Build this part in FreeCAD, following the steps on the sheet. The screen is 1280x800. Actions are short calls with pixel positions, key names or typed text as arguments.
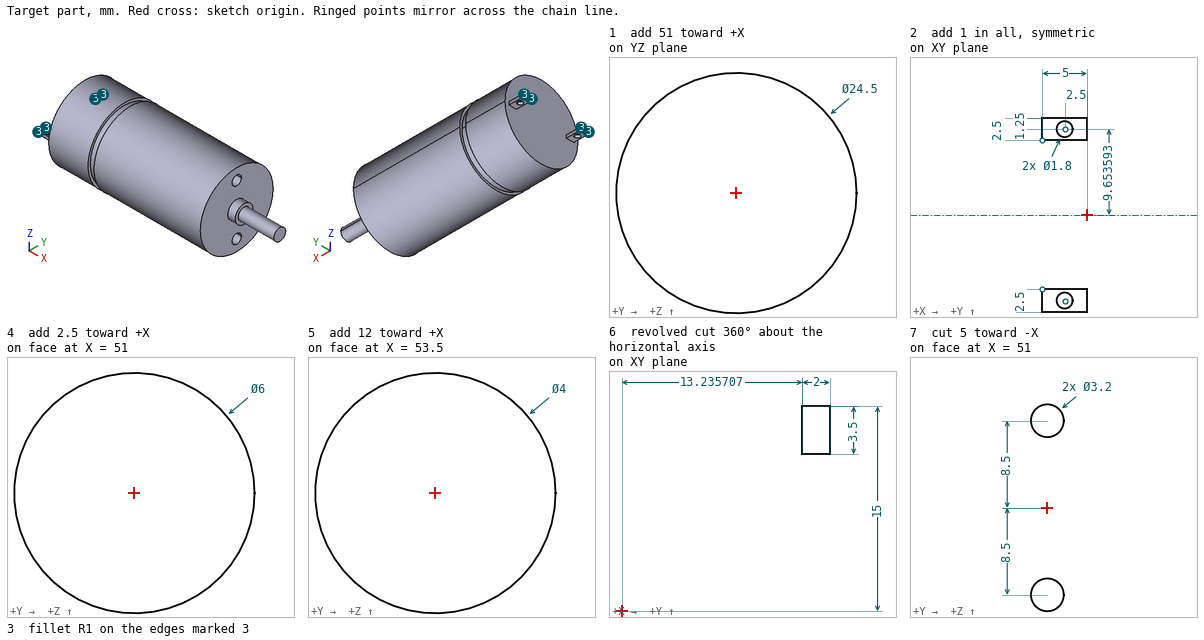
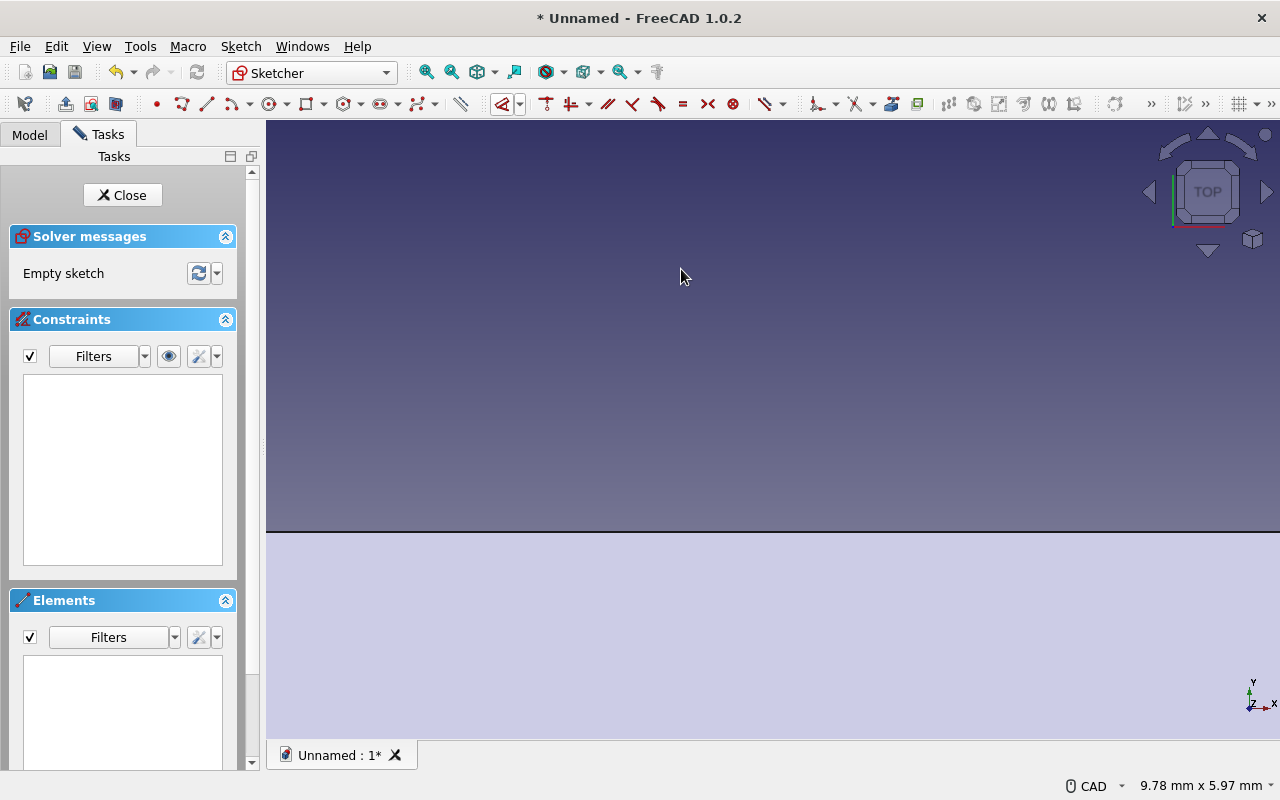
click(306, 104)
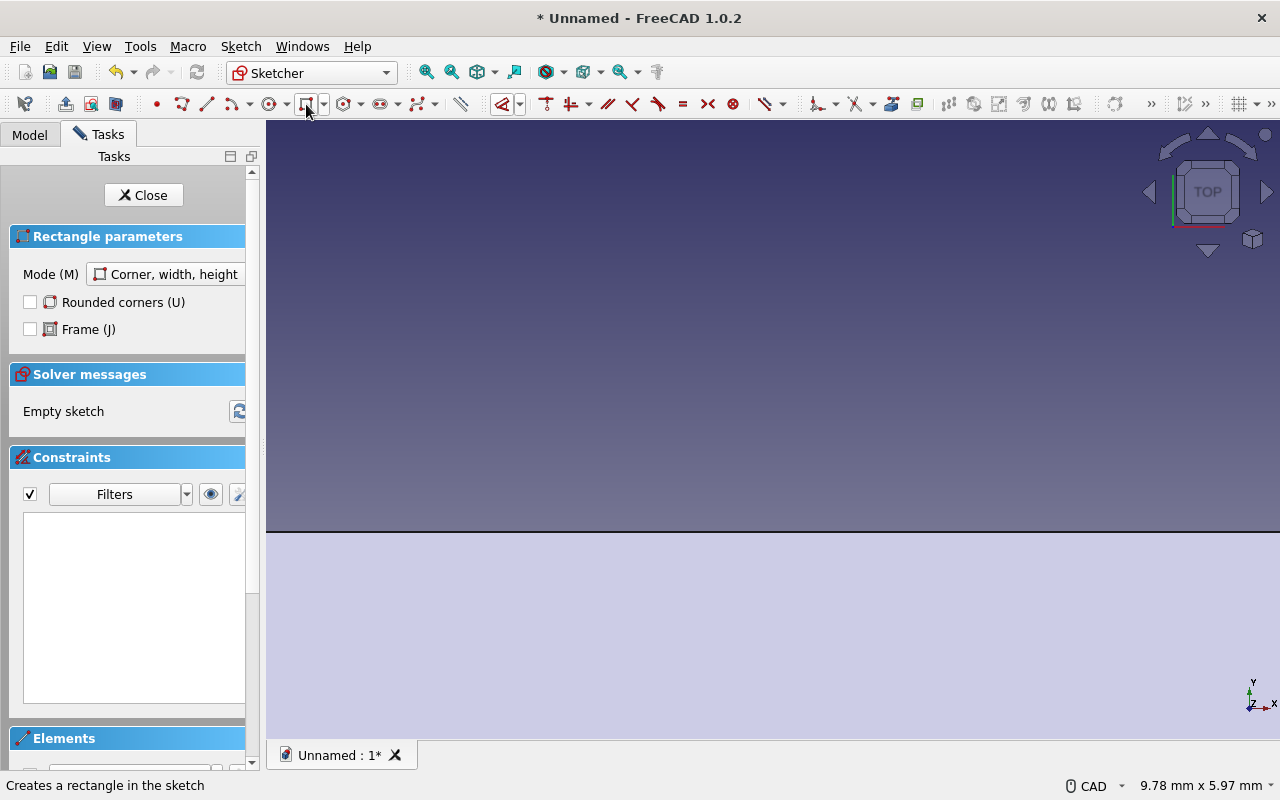
click(596, 246)
move(804, 609)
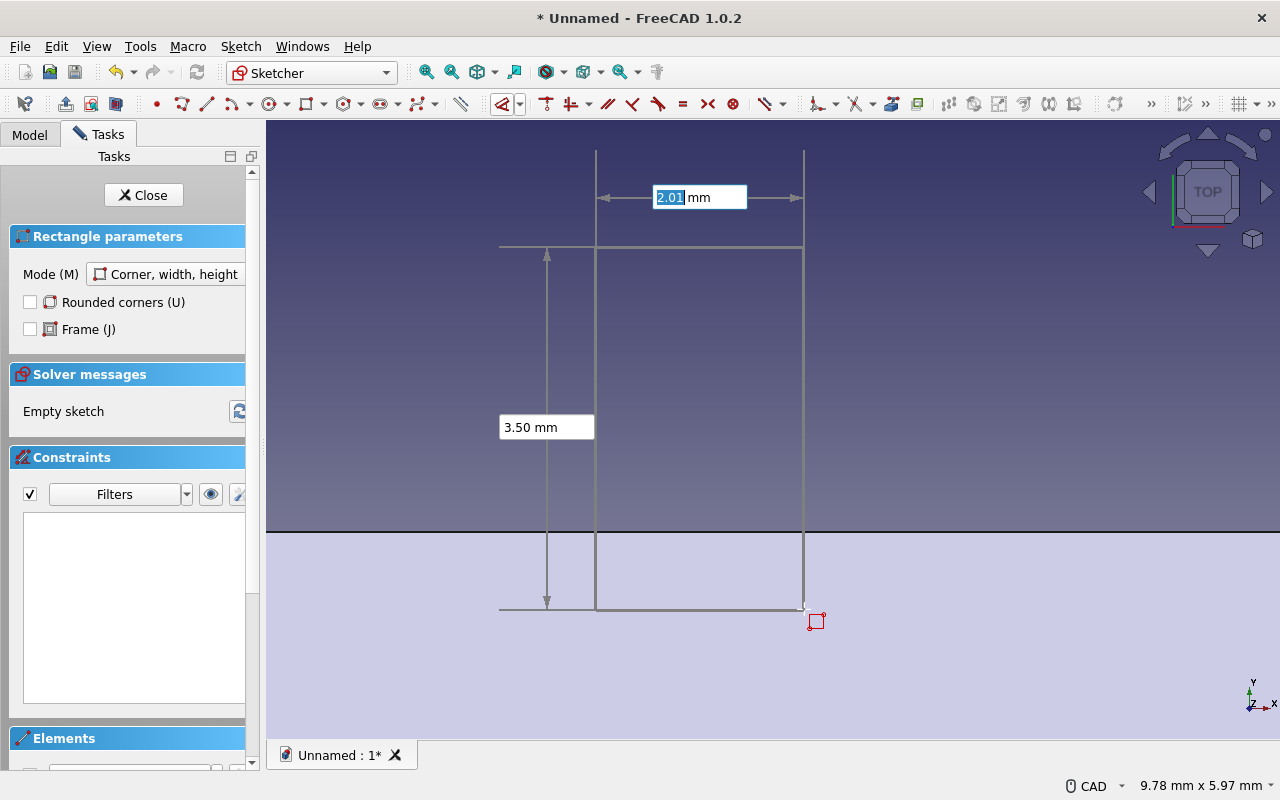
text(2)
key(Tab)
text(3.5)
key(Return)
key(Escape)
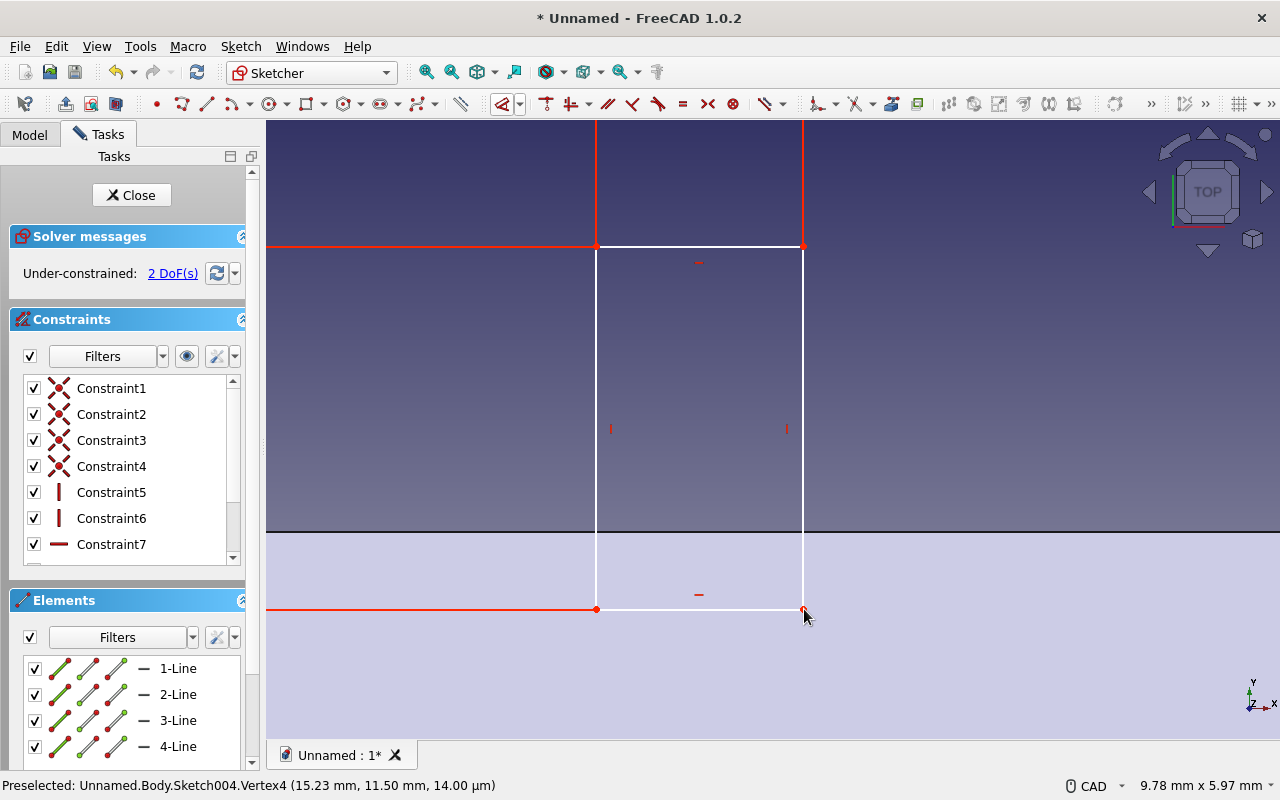
click(596, 247)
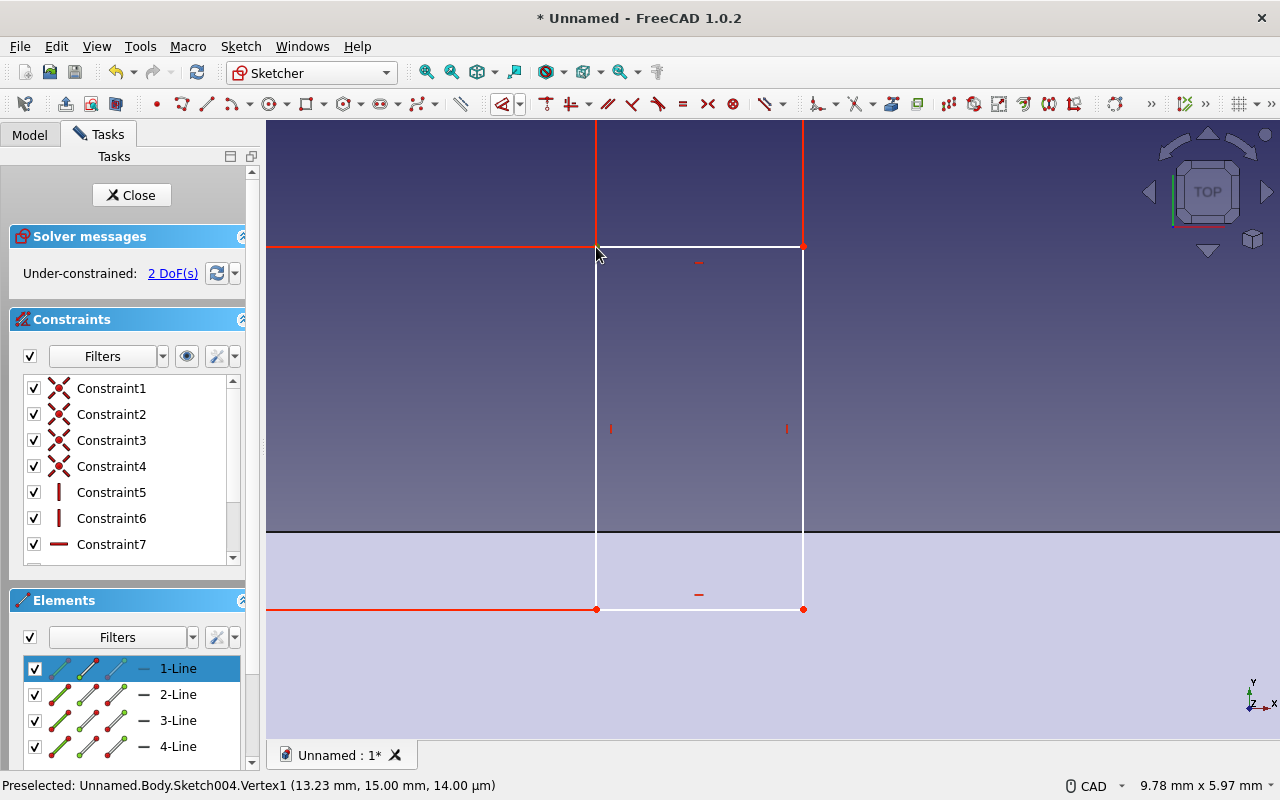
click(520, 104)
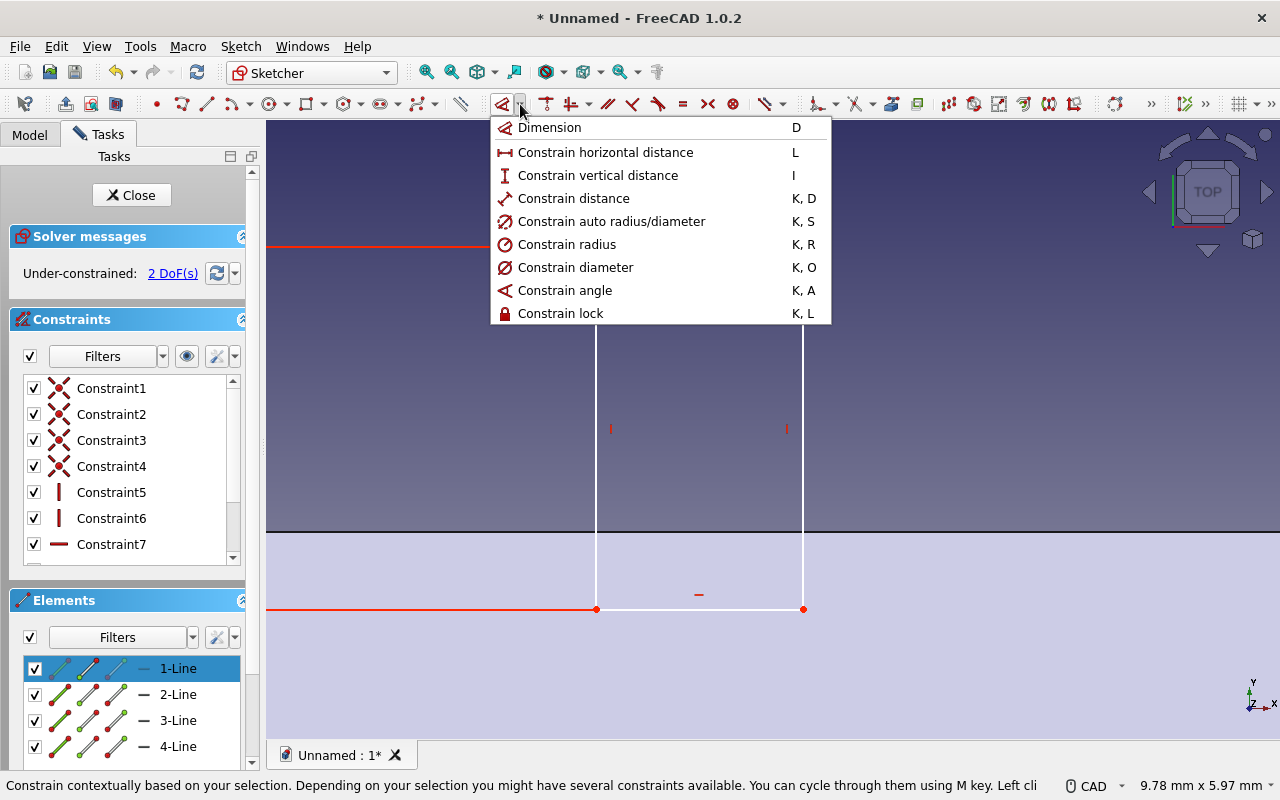
click(661, 176)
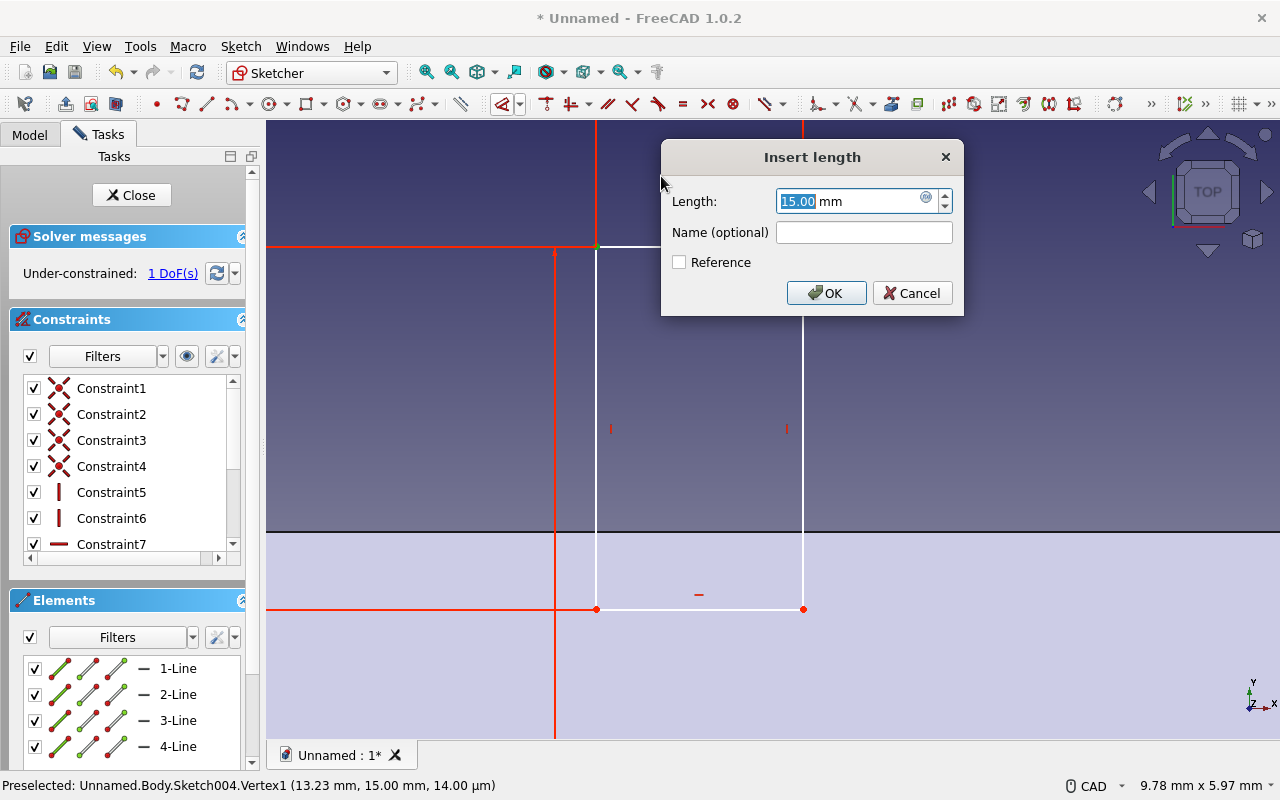
text(15)
key(Return)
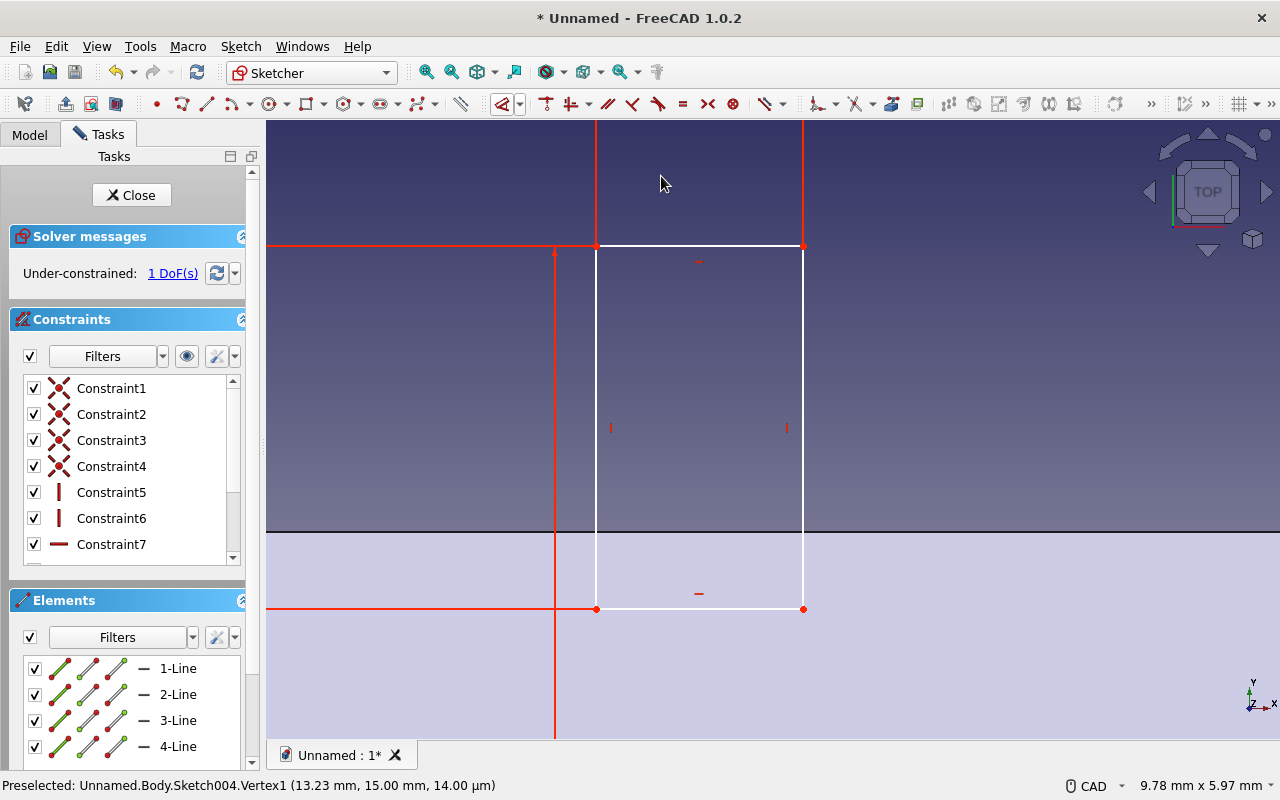
click(596, 246)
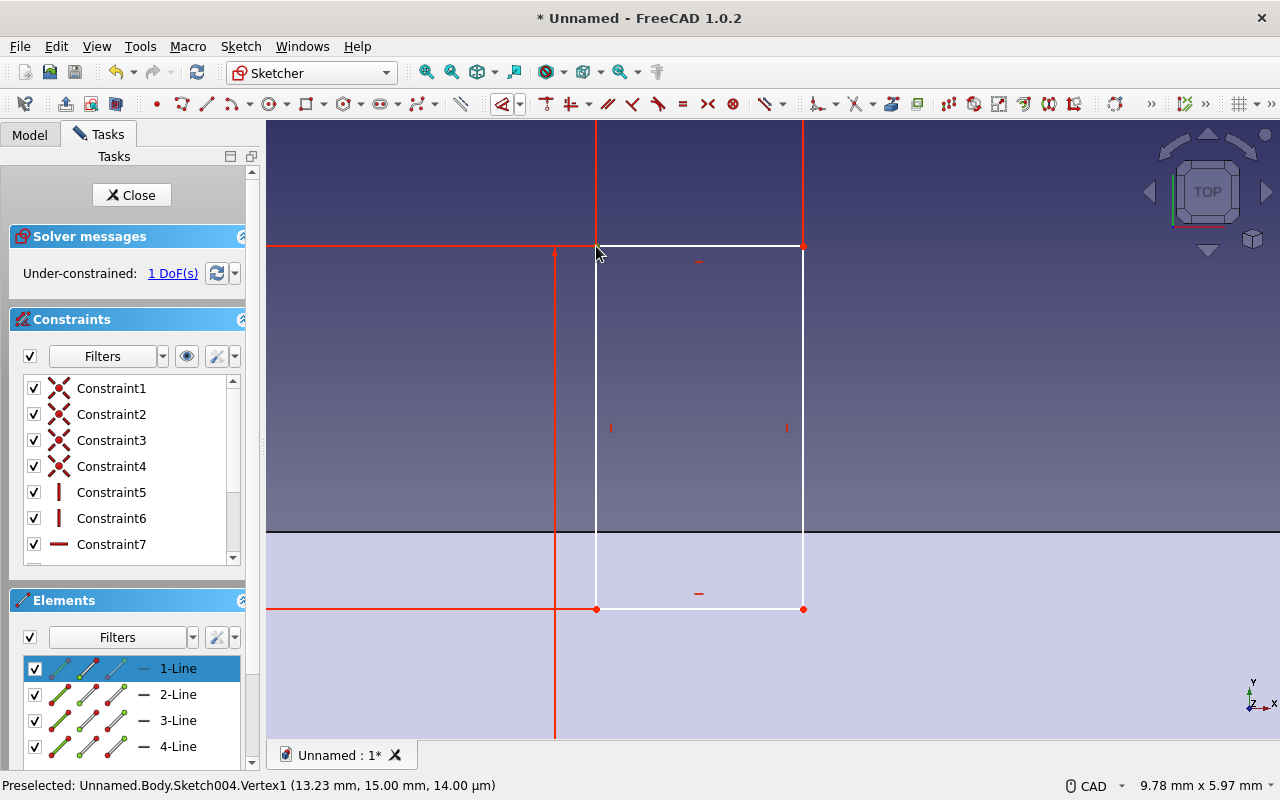
click(520, 104)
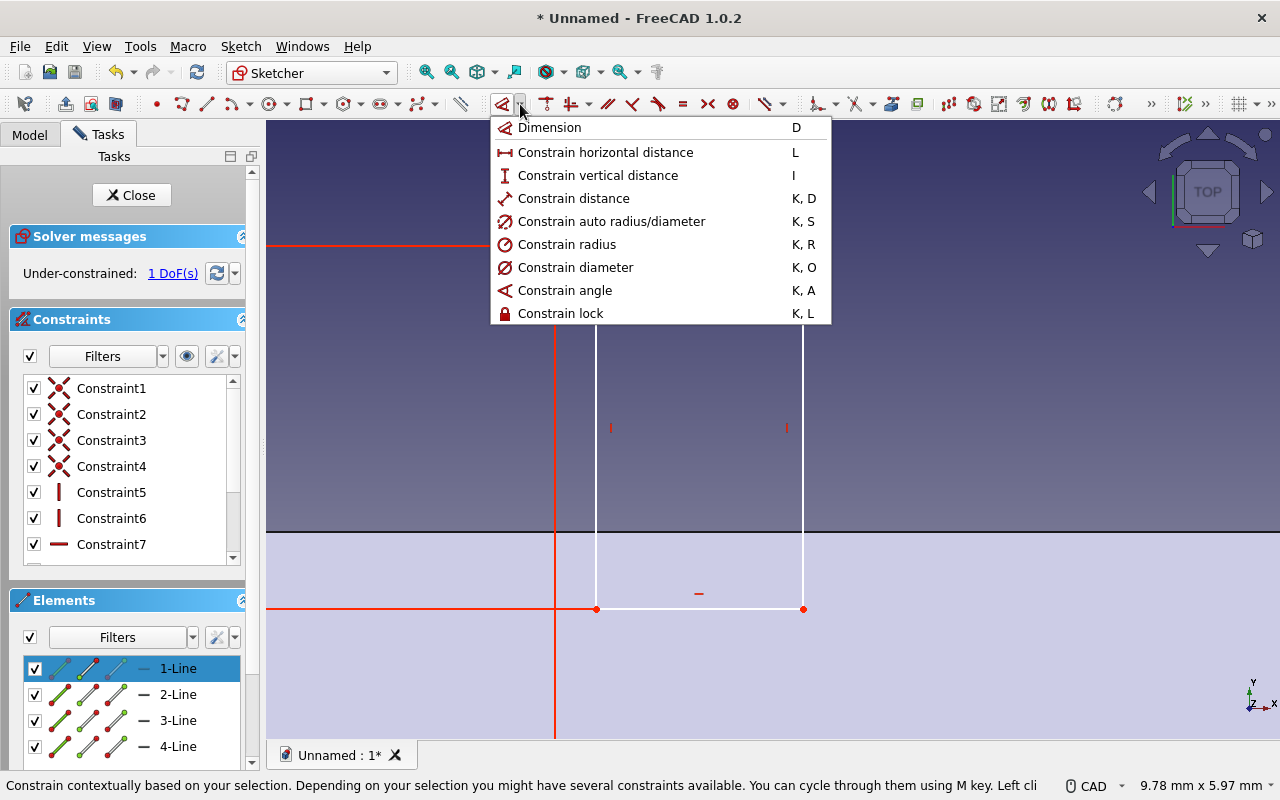
click(661, 152)